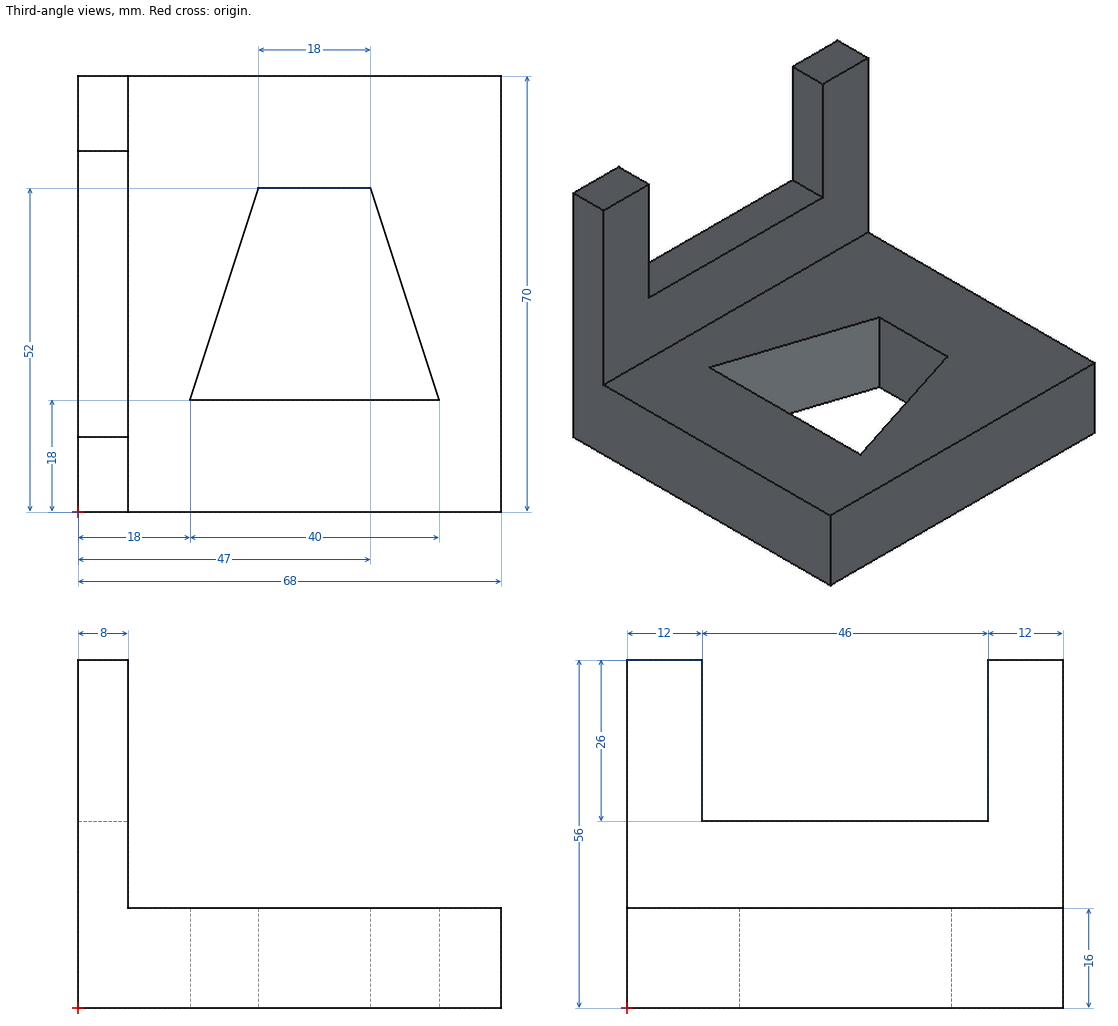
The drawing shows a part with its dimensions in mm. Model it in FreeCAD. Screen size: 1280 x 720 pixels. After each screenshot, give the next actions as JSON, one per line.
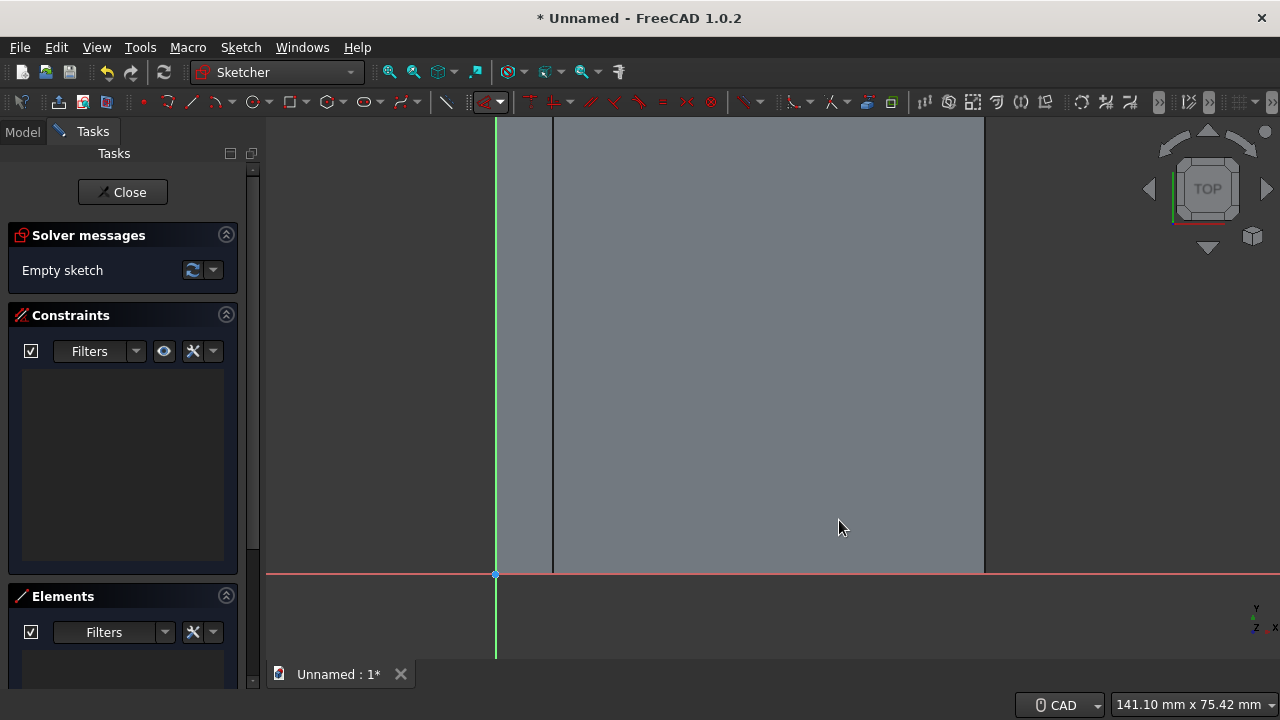
{"action": "key", "text": "g m"}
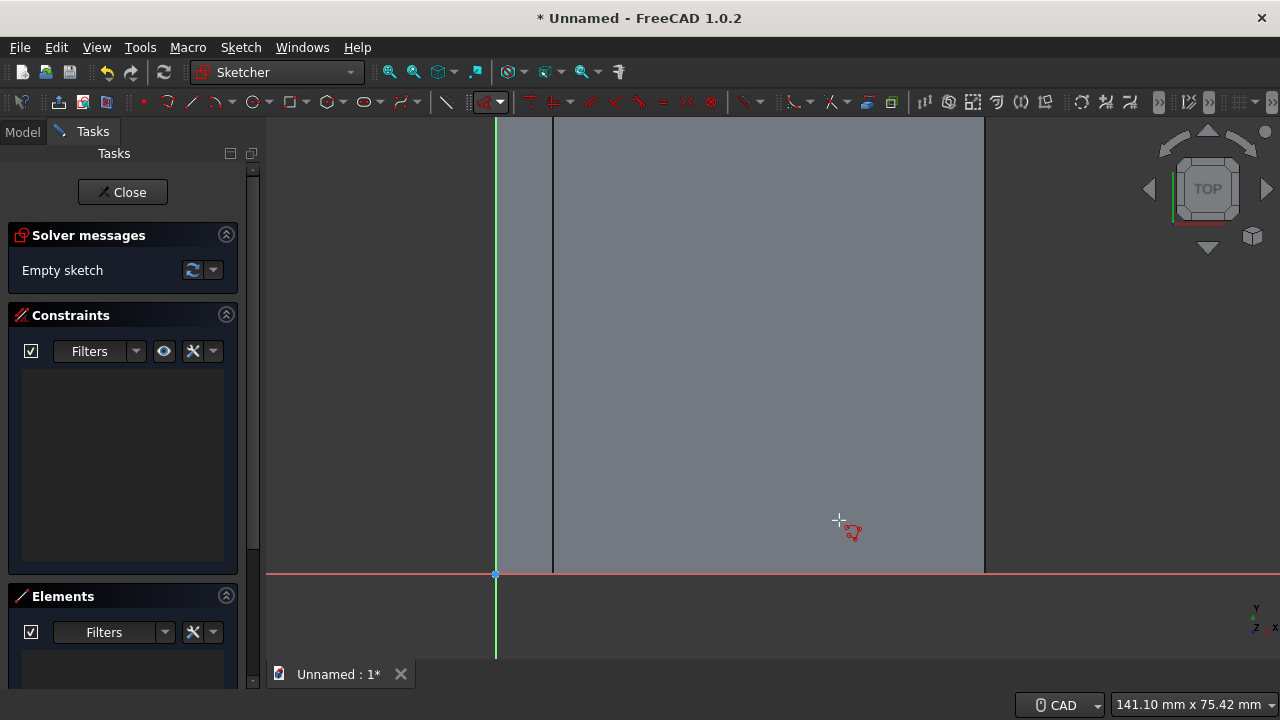
{"action": "left_click", "coordinate": [625, 445]}
{"action": "left_click", "coordinate": [913, 445]}
{"action": "left_click", "coordinate": [834, 201]}
{"action": "left_click", "coordinate": [704, 201]}
{"action": "left_click", "coordinate": [625, 446]}
{"action": "key", "text": "Escape"}
{"action": "key", "text": "Escape"}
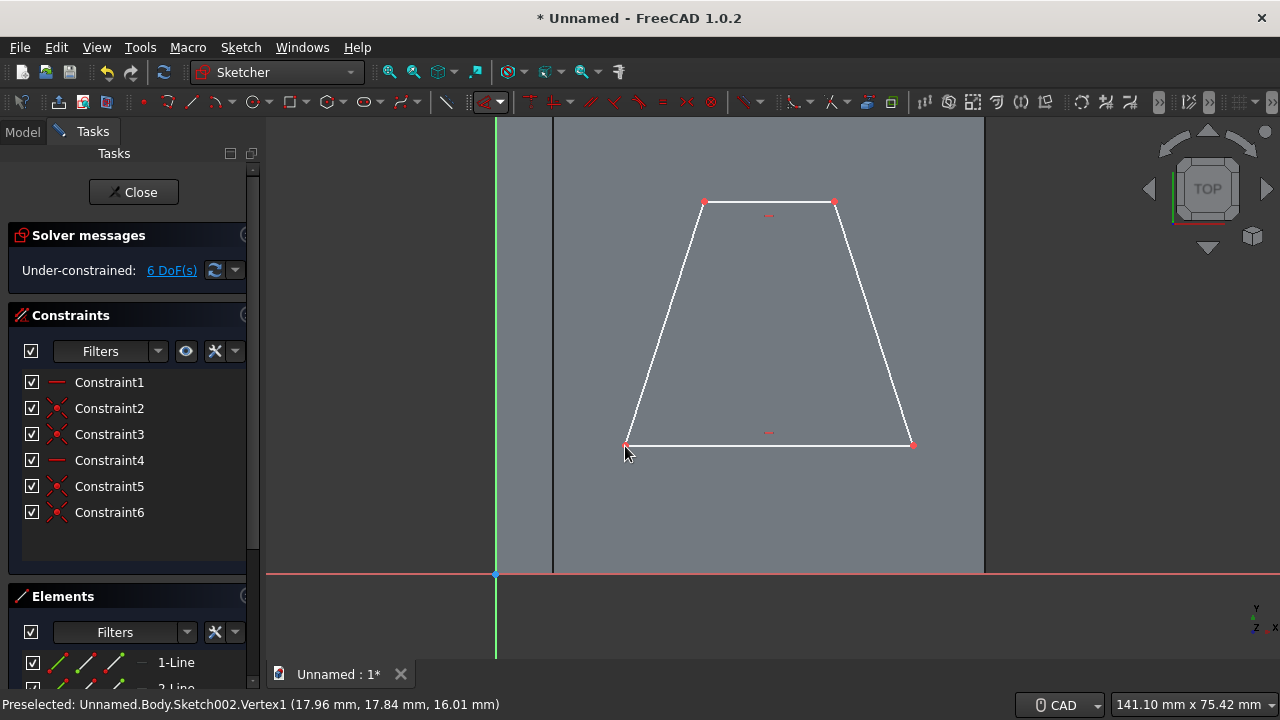
{"action": "left_click", "coordinate": [711, 446]}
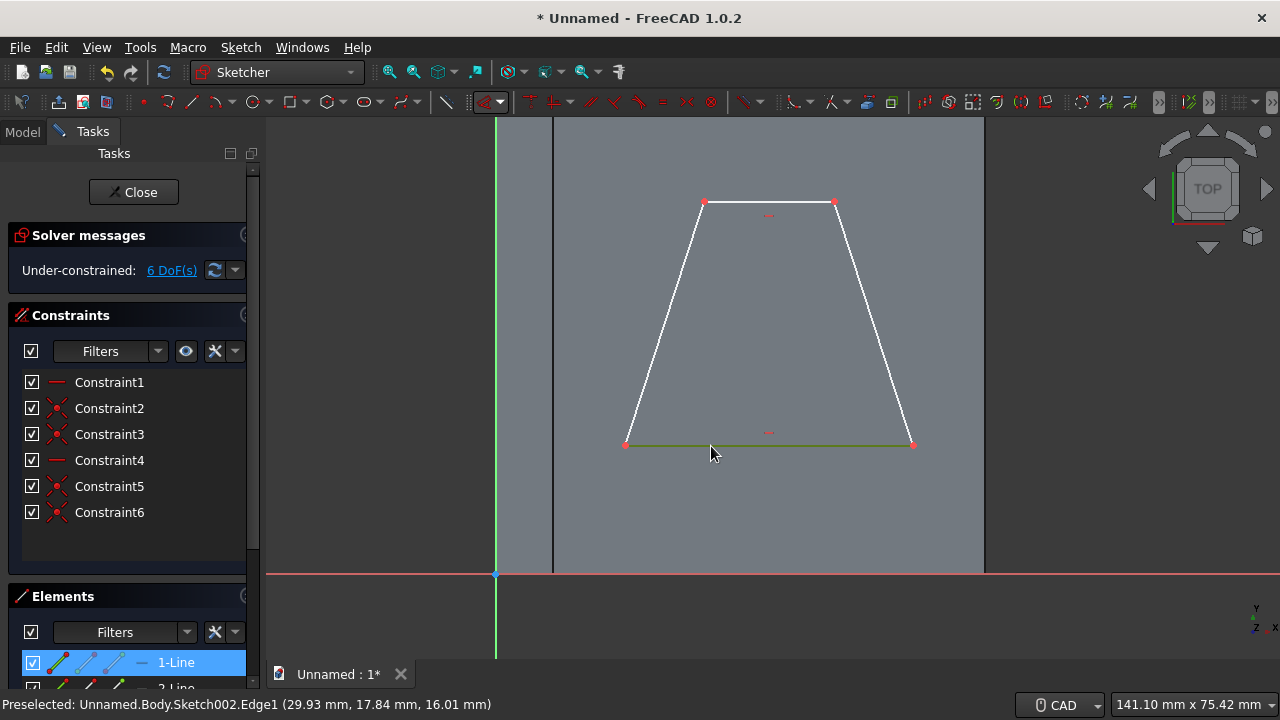
{"action": "key", "text": "l"}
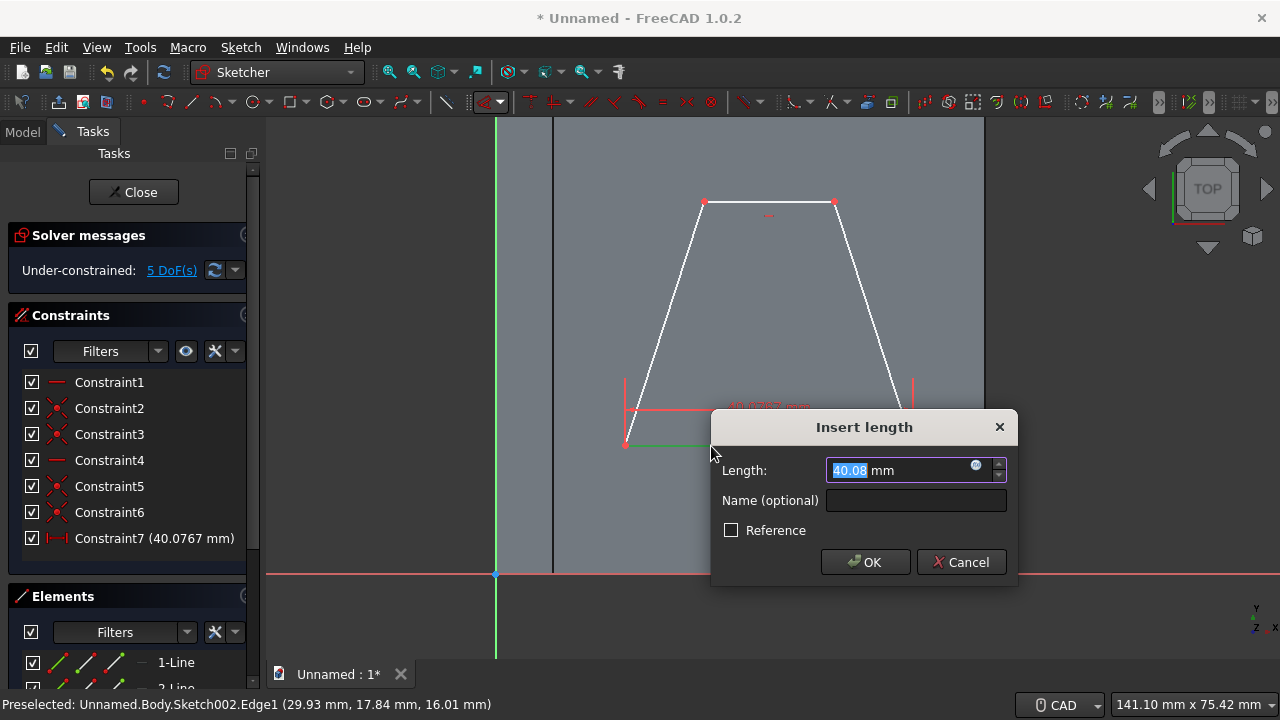
{"action": "type", "text": "40"}
{"action": "key", "text": "Return"}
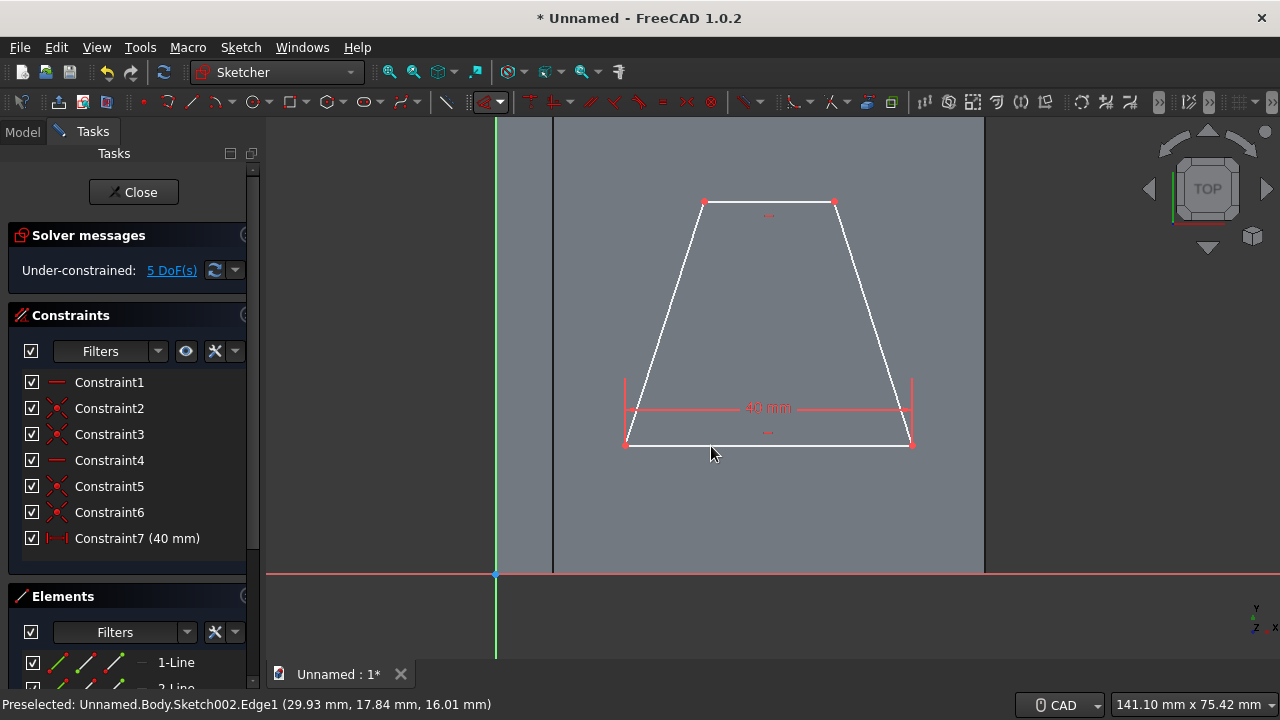
{"action": "left_click", "coordinate": [795, 202]}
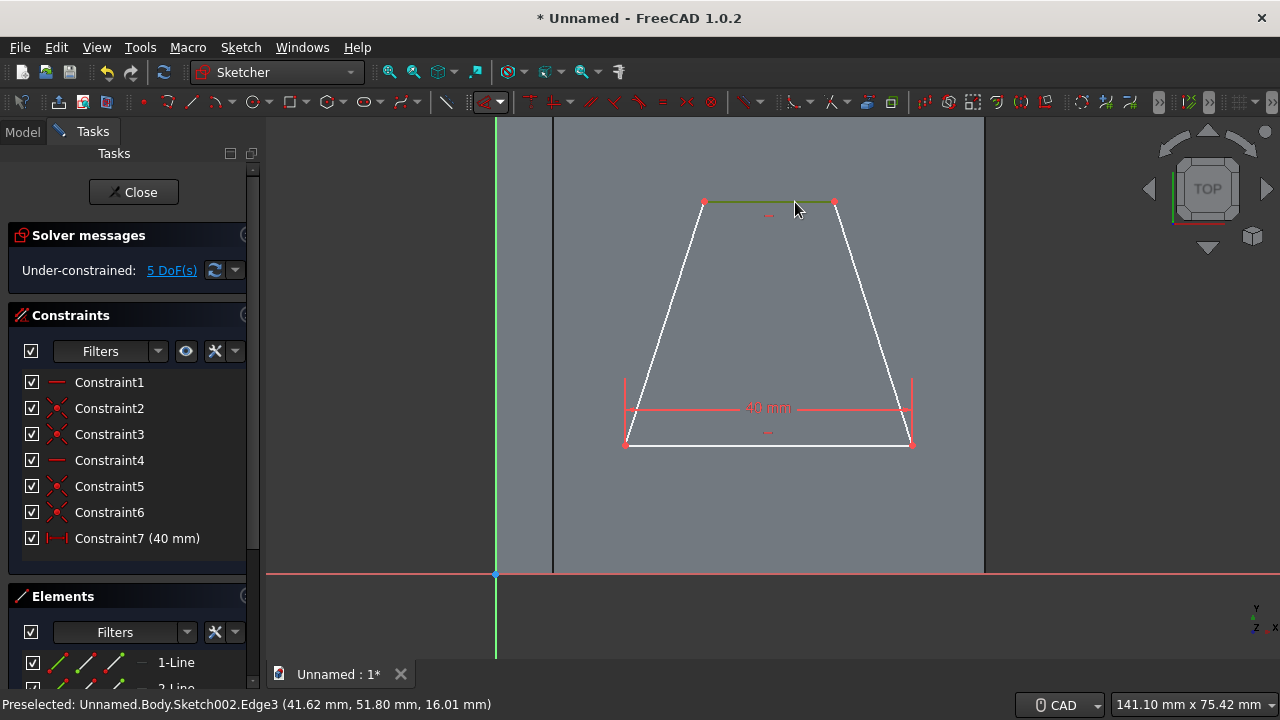
{"action": "key", "text": "l"}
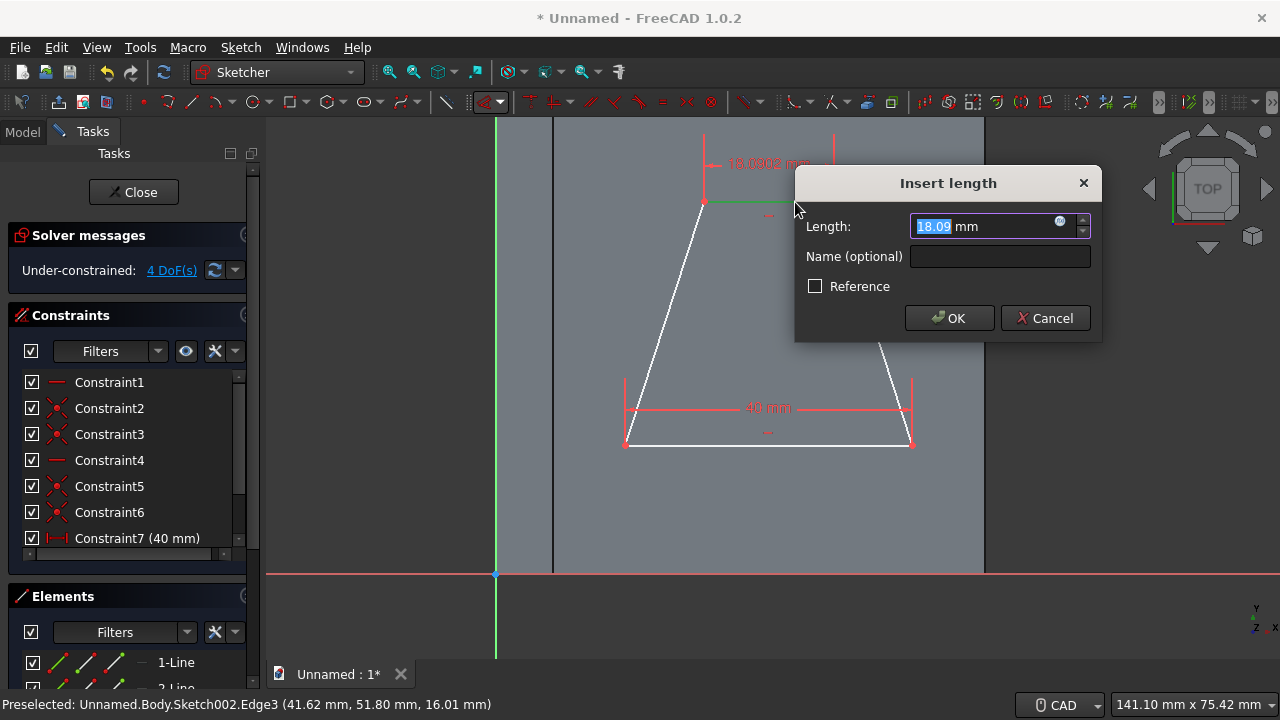
{"action": "type", "text": "18"}
{"action": "key", "text": "Return"}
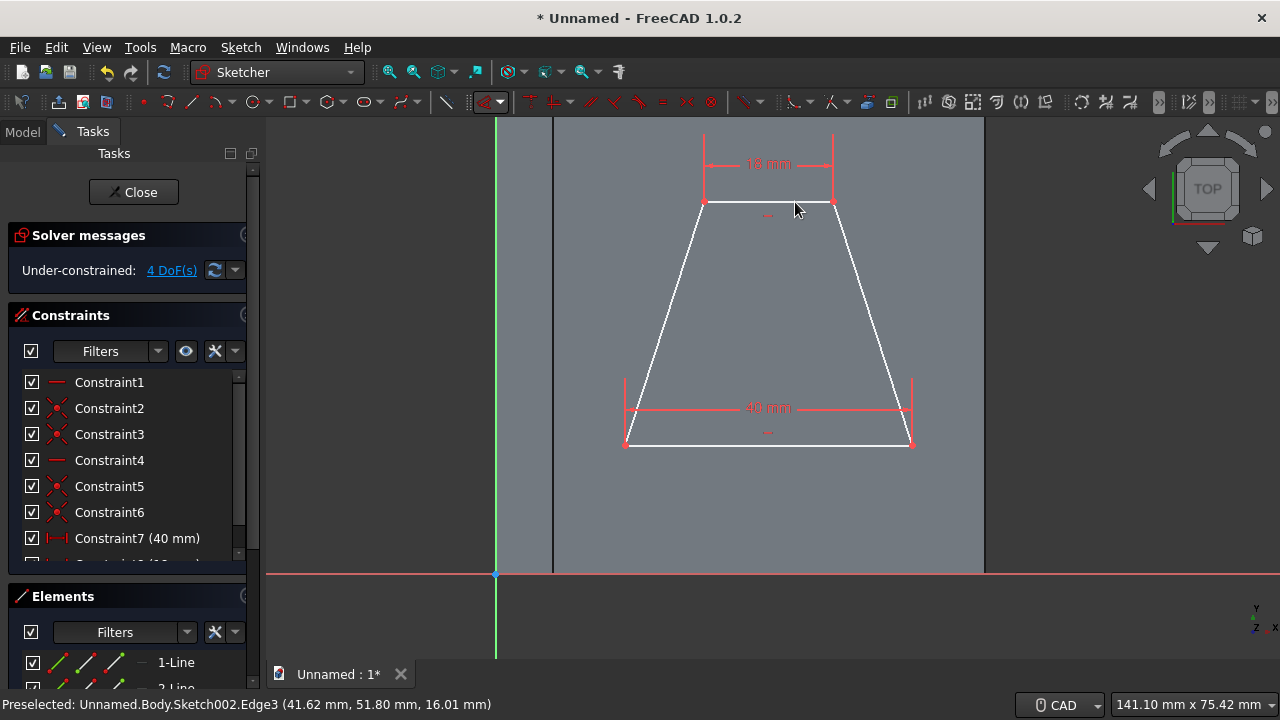
{"action": "left_click", "coordinate": [625, 446]}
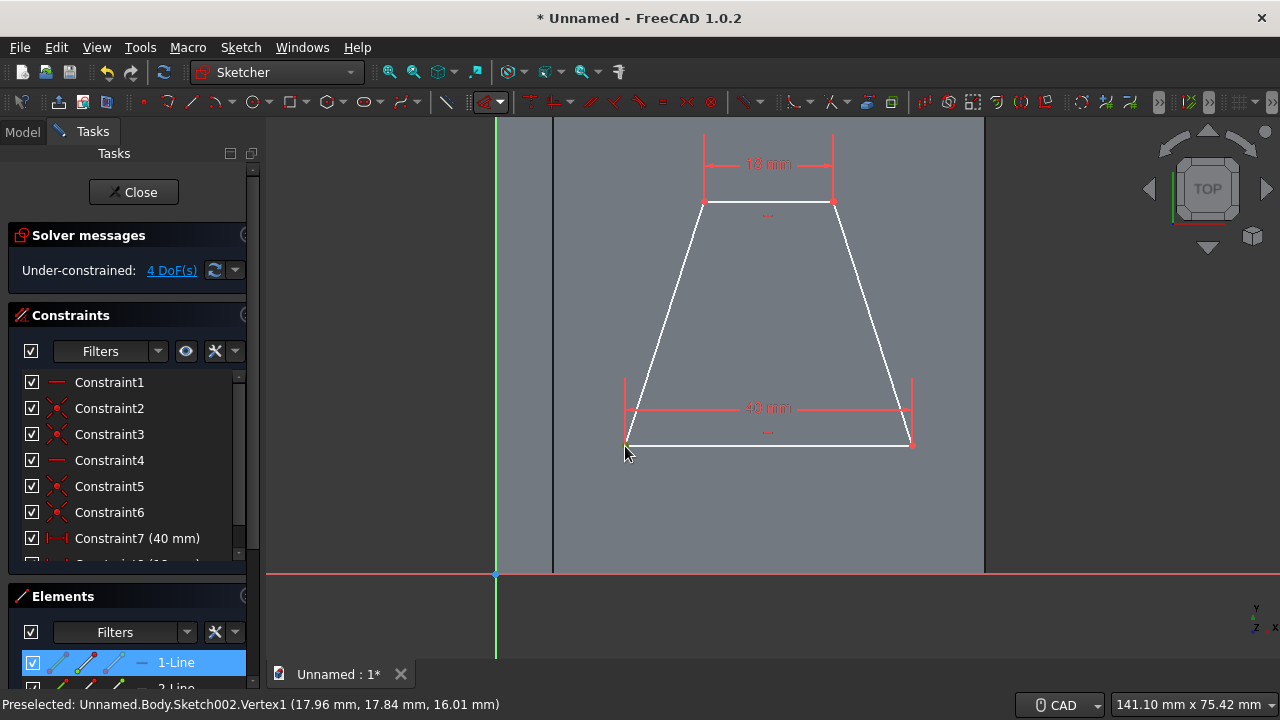
{"action": "left_click", "coordinate": [502, 102]}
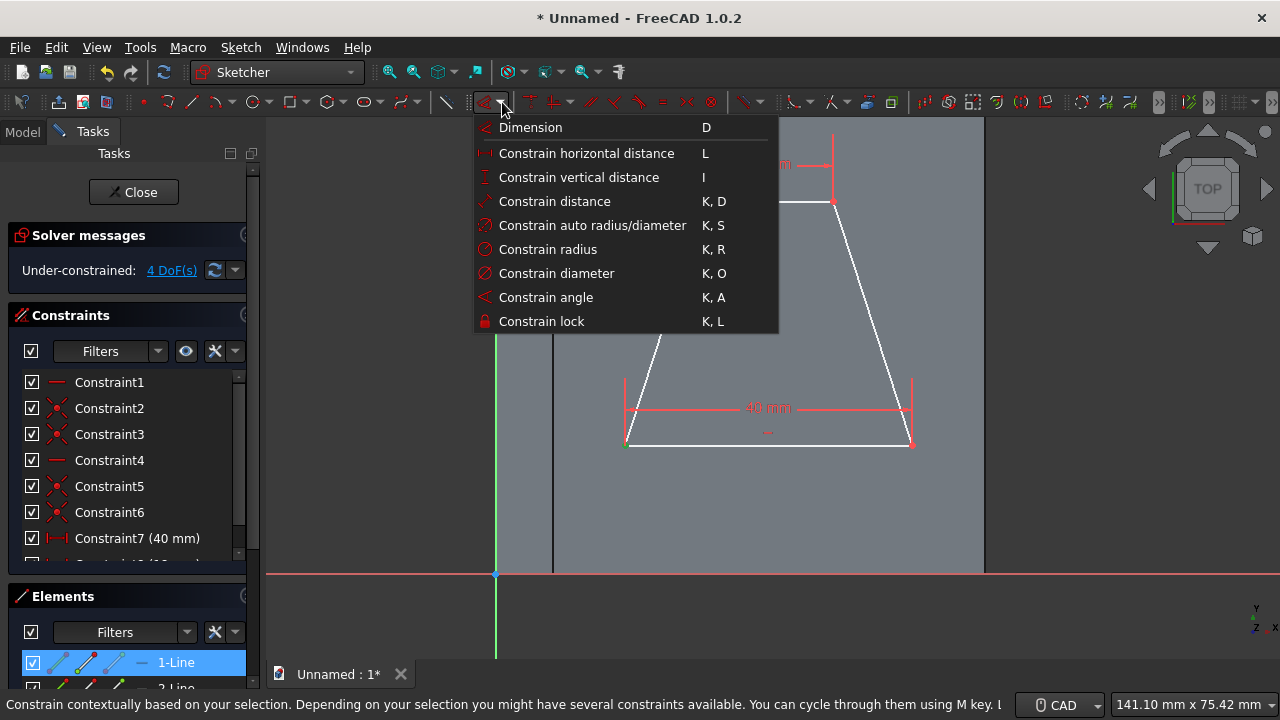
{"action": "left_click", "coordinate": [626, 153]}